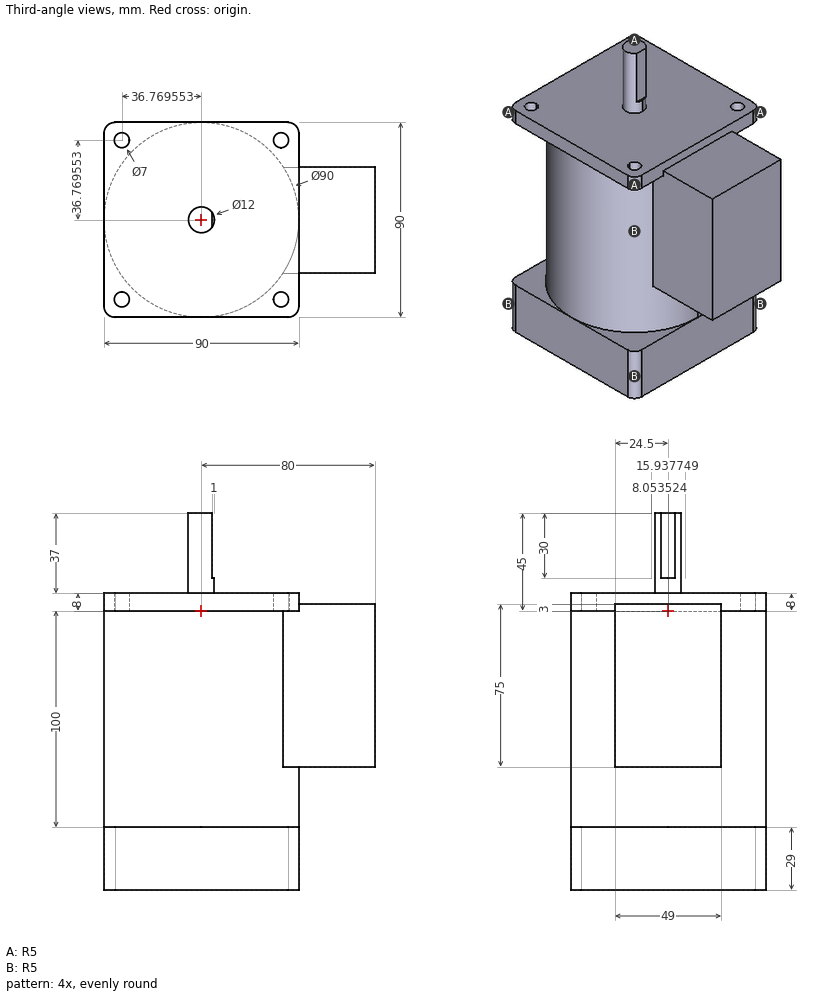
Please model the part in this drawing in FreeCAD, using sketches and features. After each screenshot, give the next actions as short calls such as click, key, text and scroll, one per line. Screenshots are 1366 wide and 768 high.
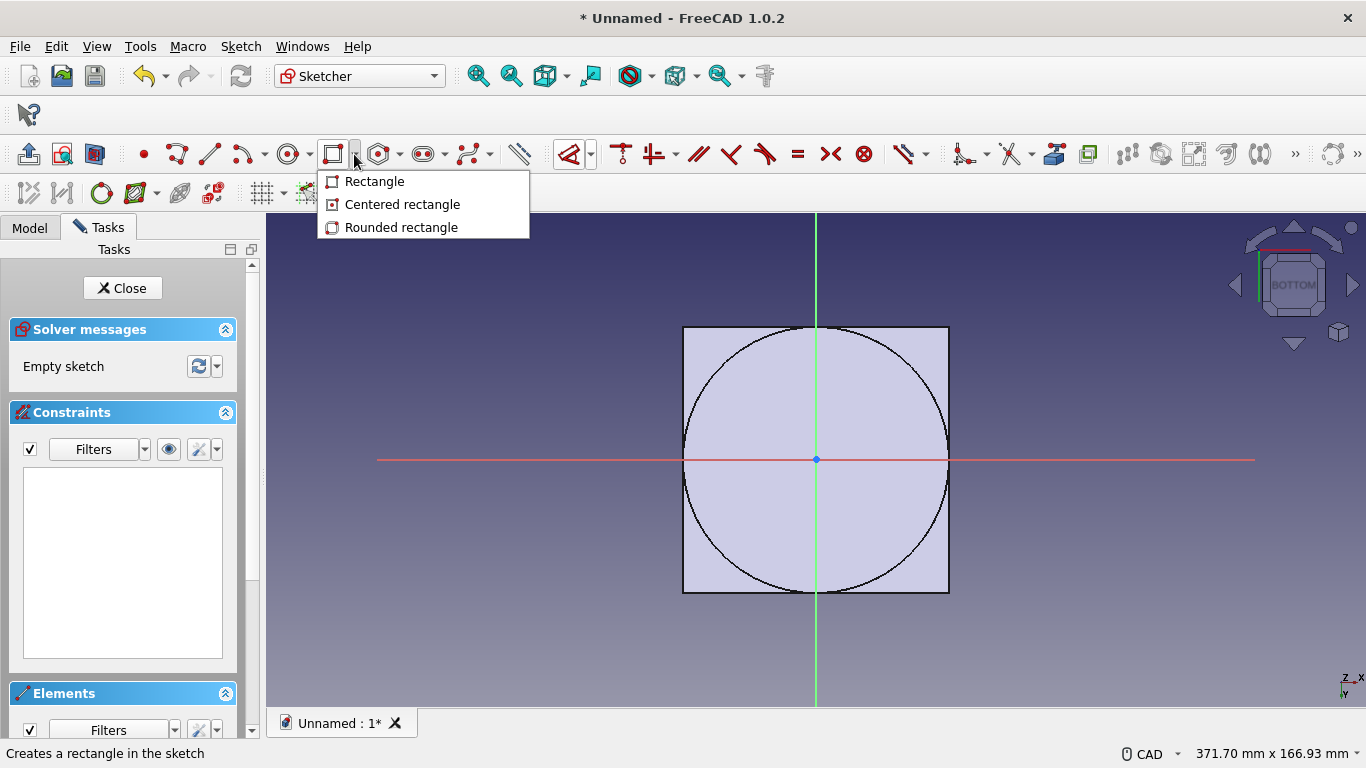
click(424, 204)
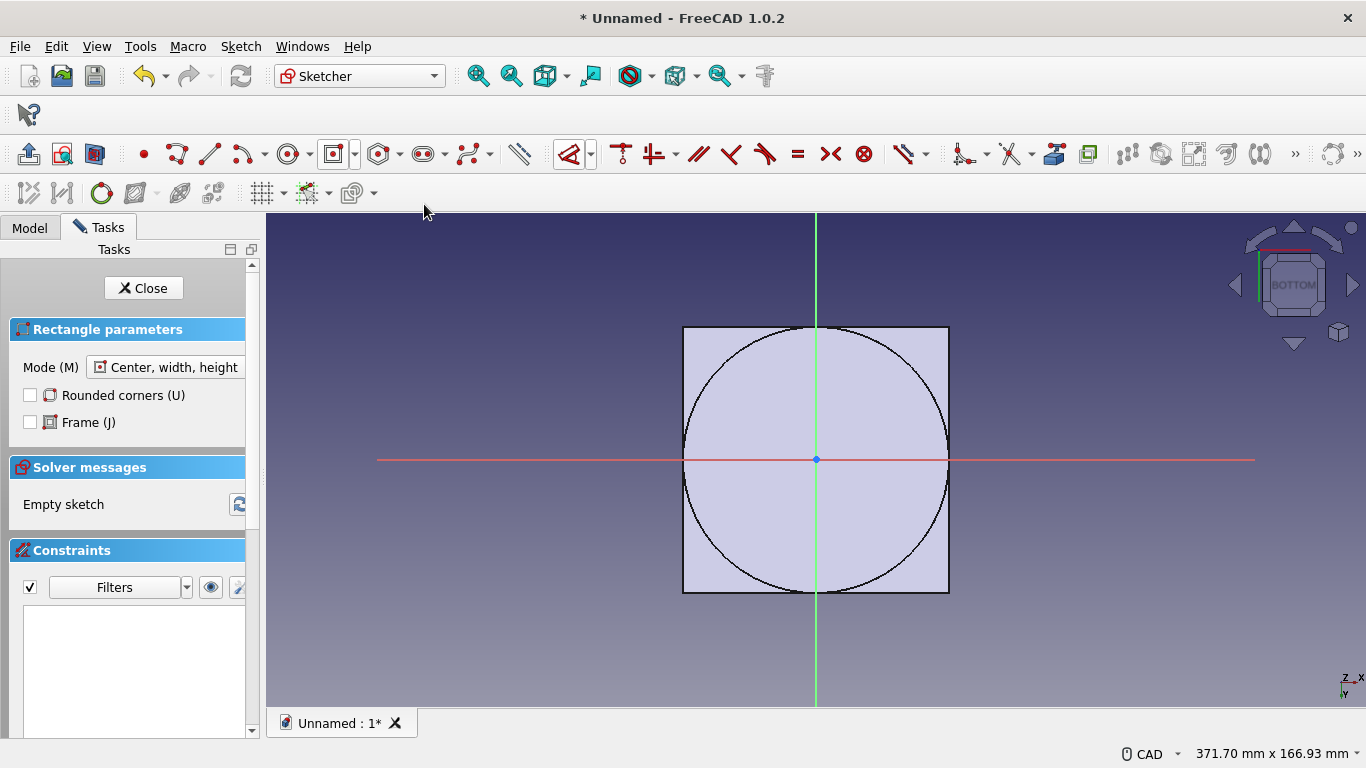
click(816, 460)
click(949, 327)
key(Escape)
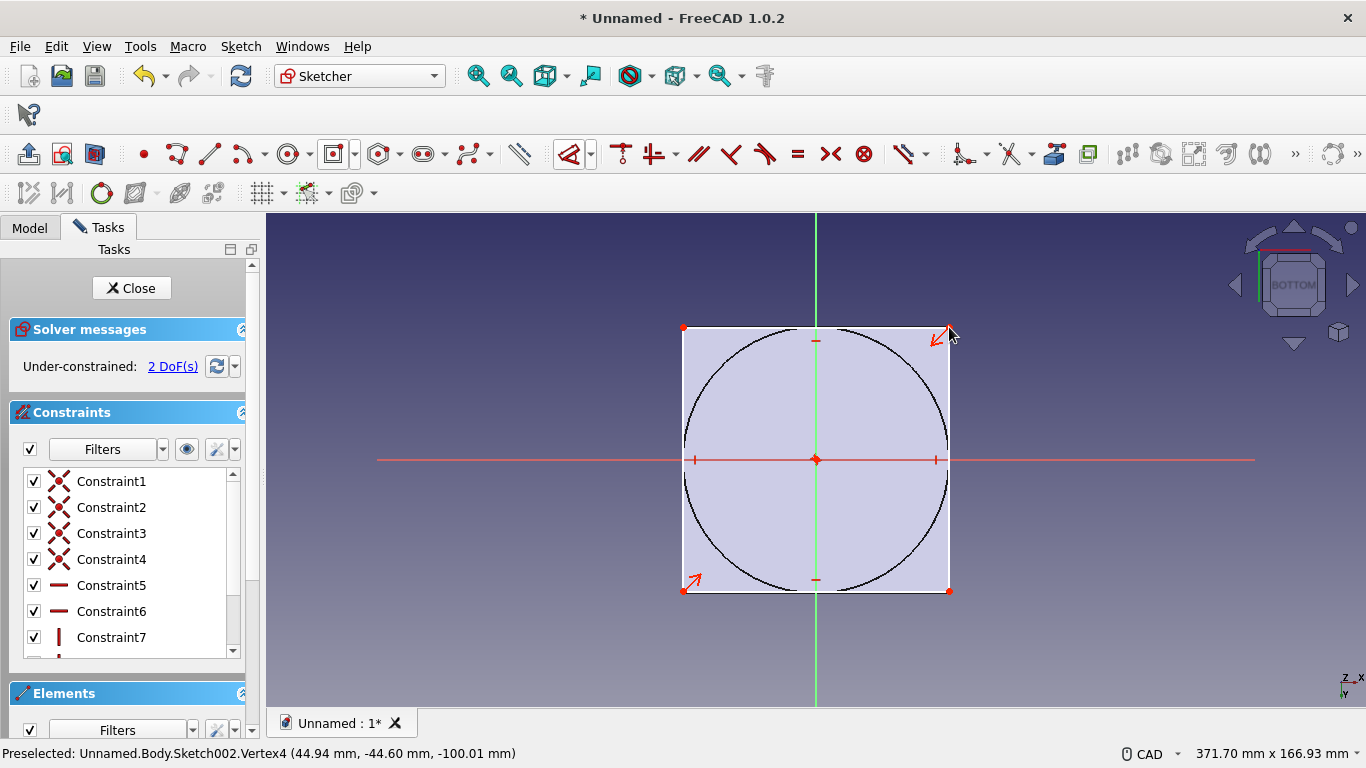
click(763, 592)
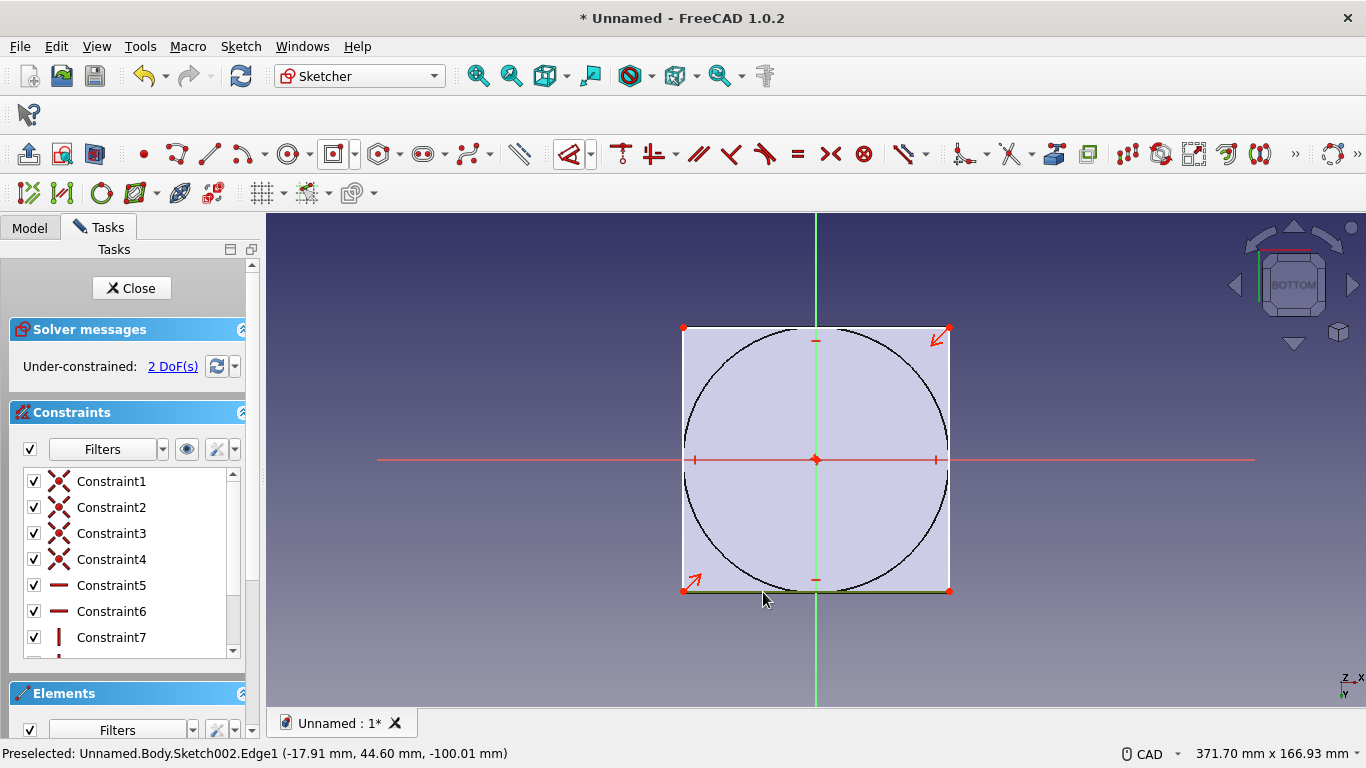
key(l)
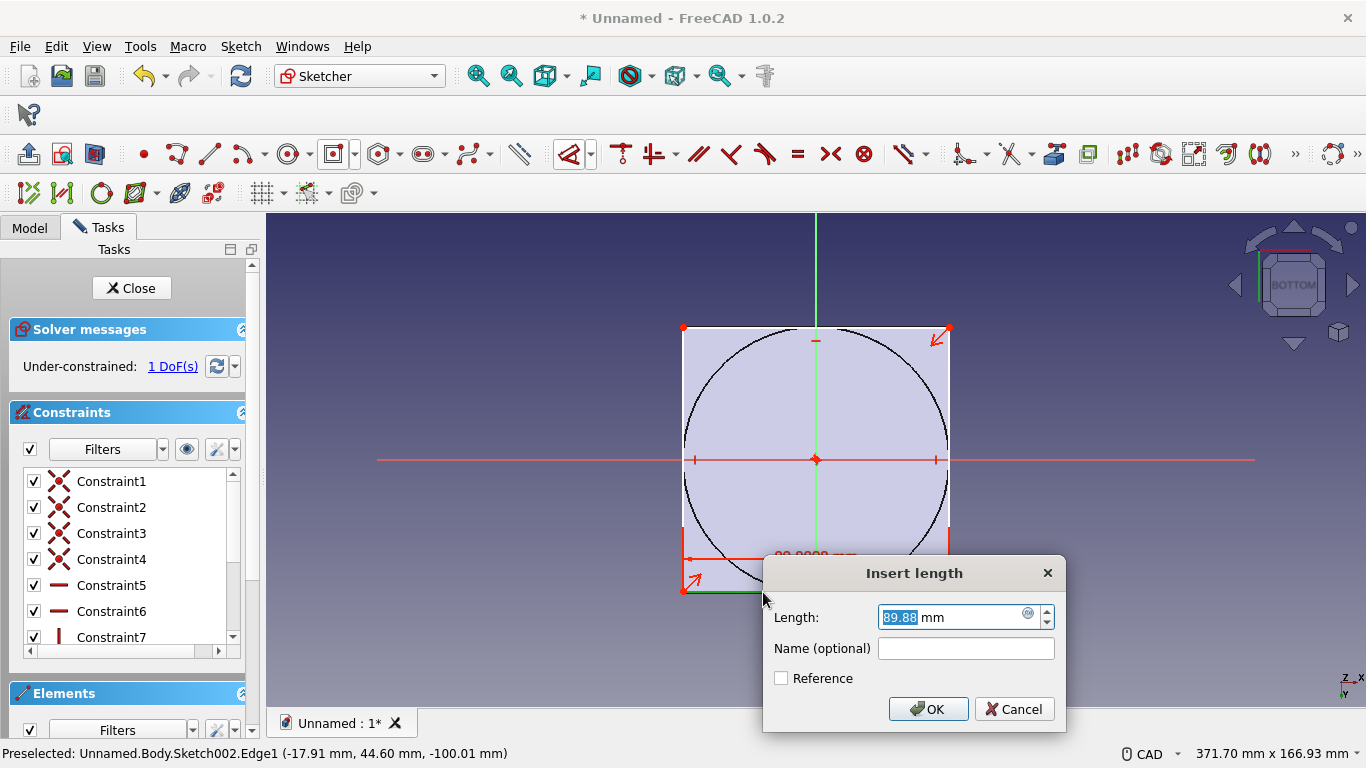
text(90)
key(Return)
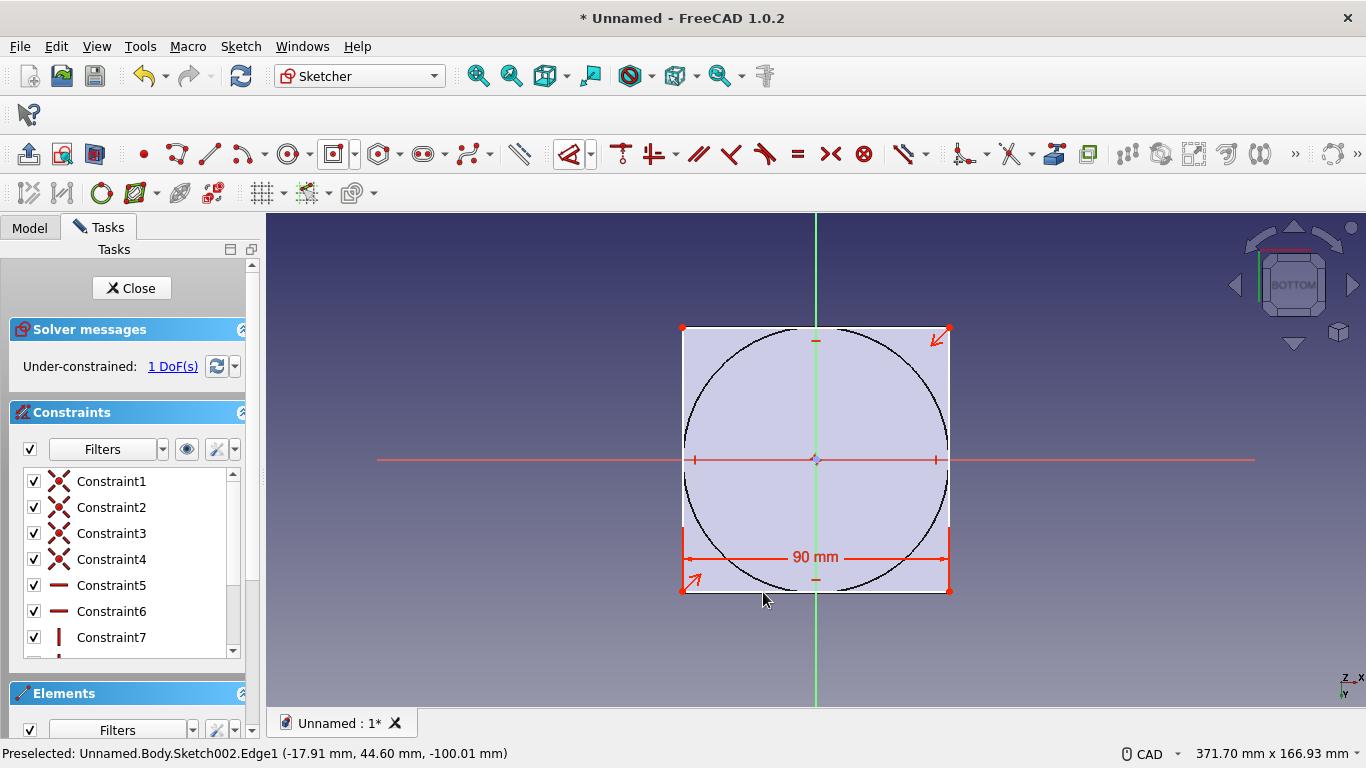
click(949, 513)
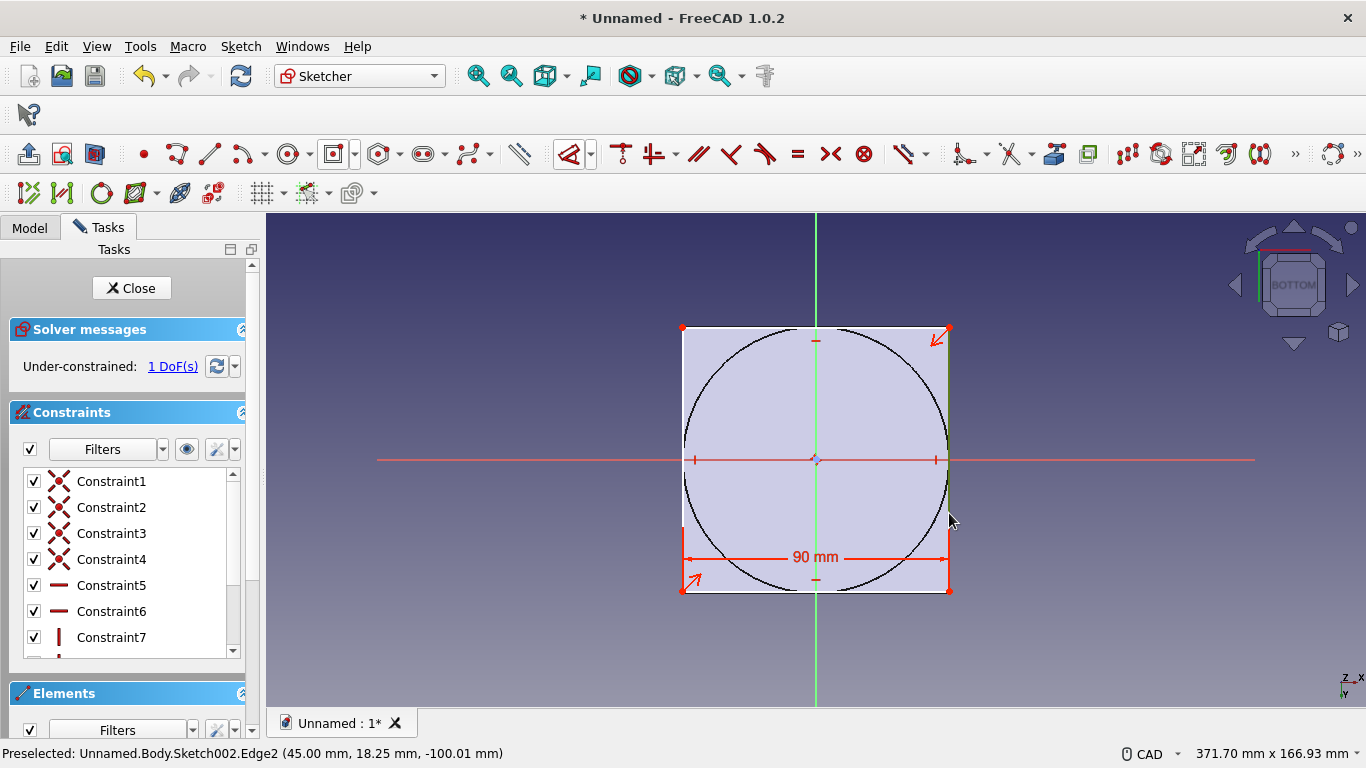
click(590, 154)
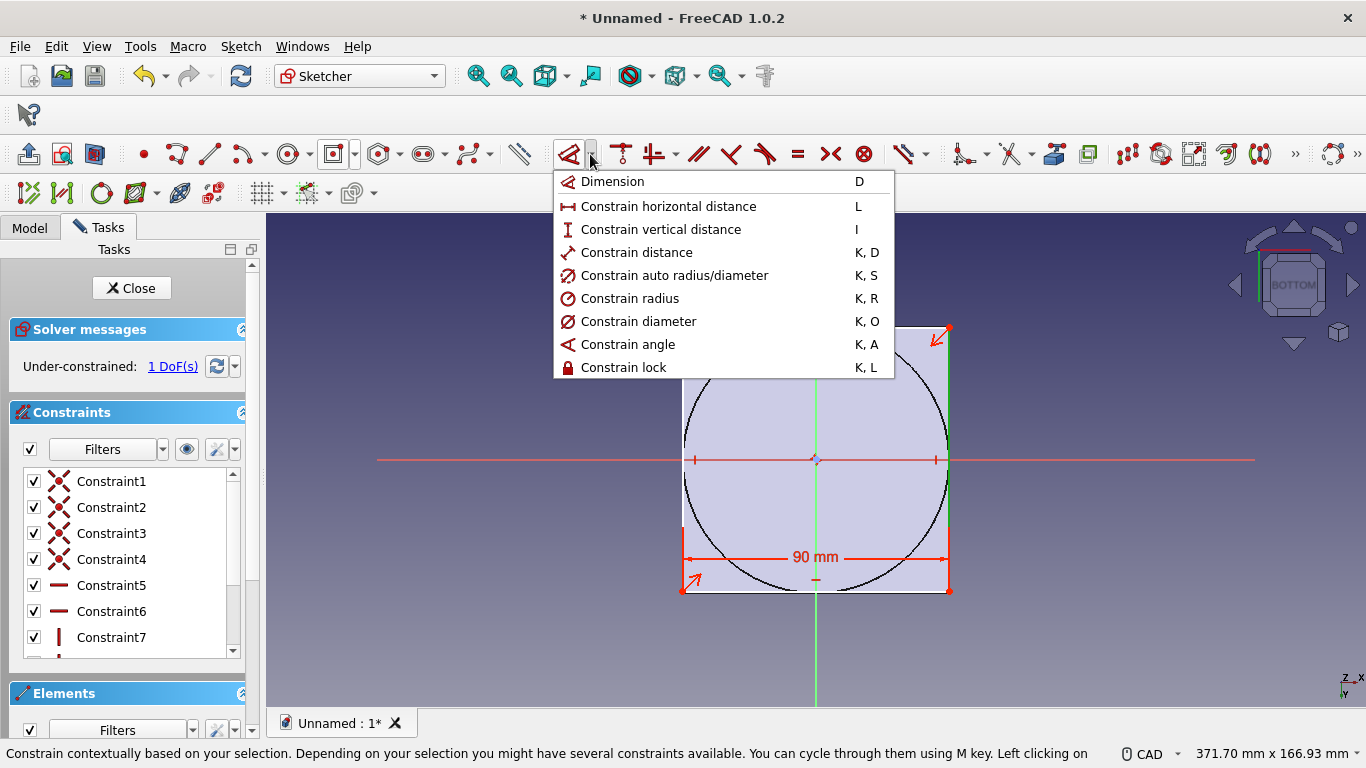
click(724, 230)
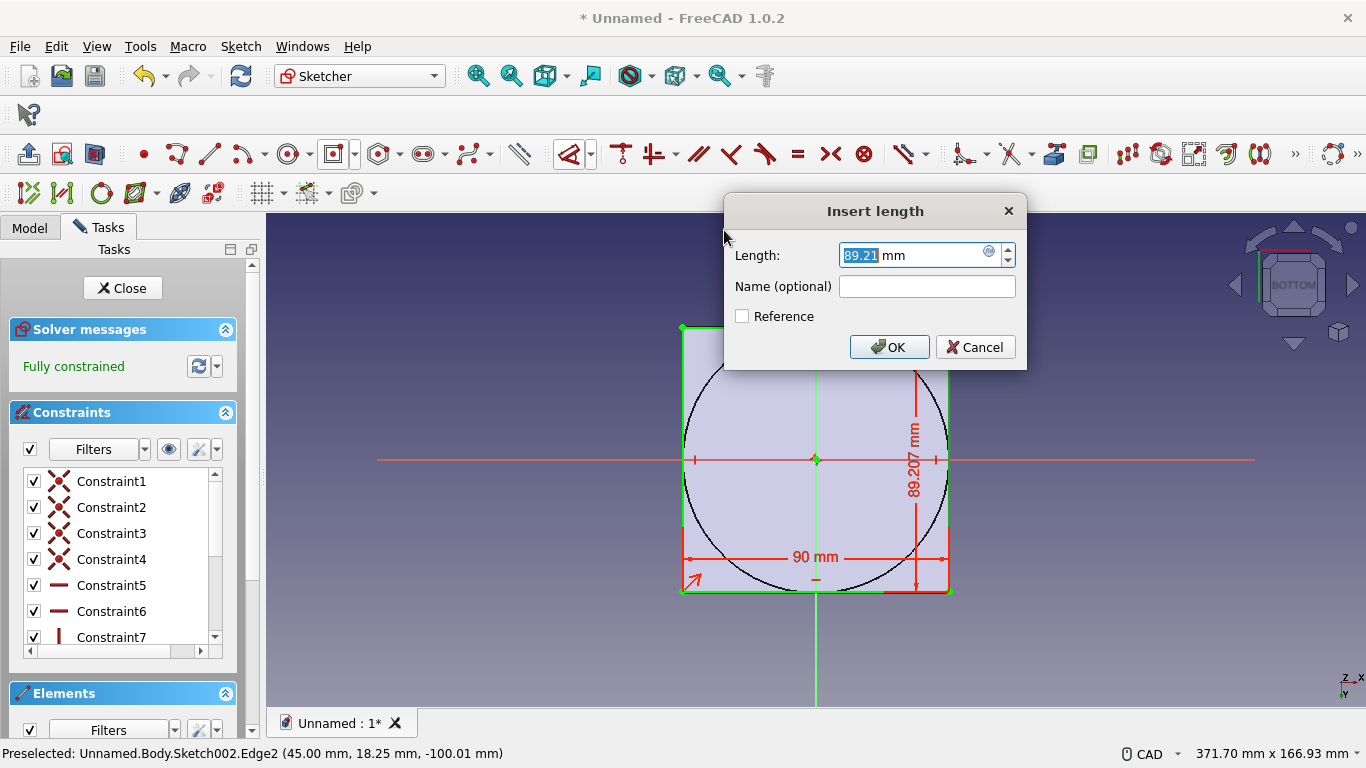
text(90)
key(Return)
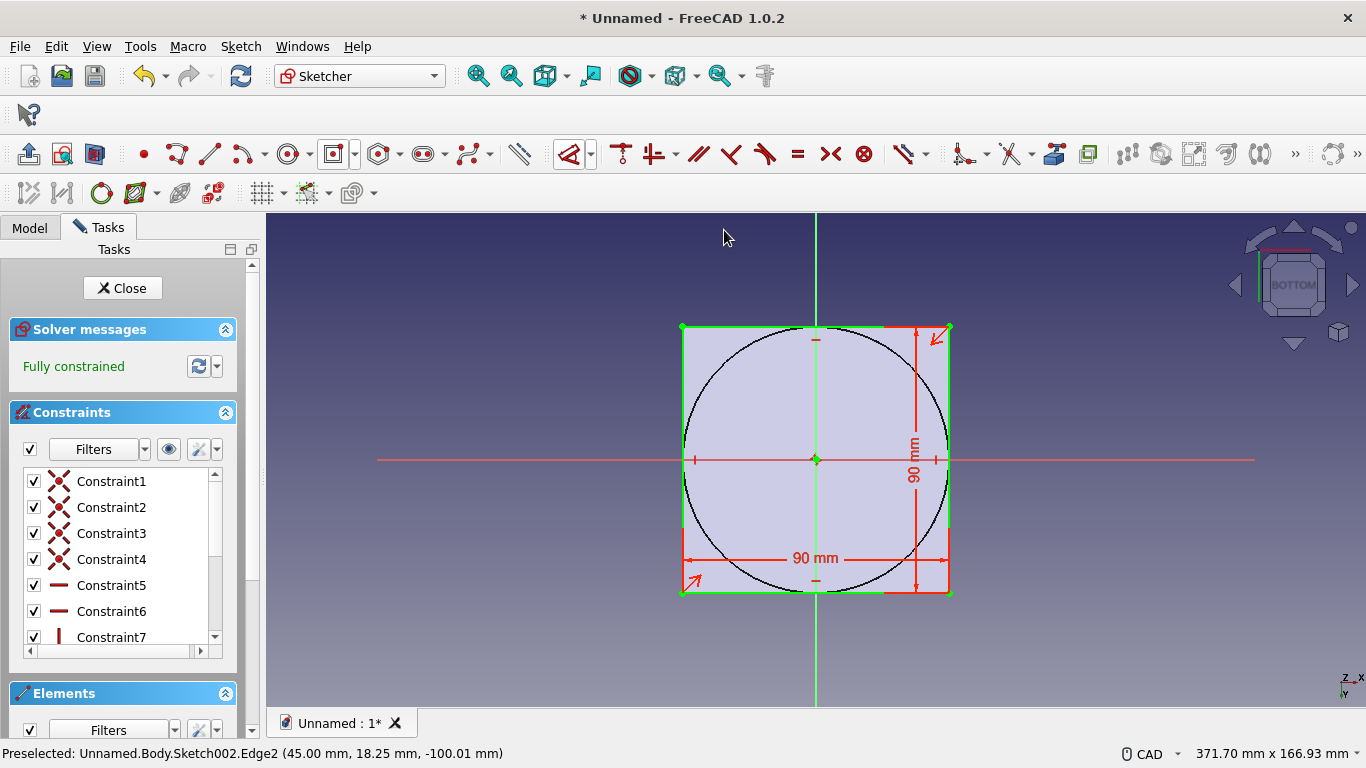
click(123, 288)